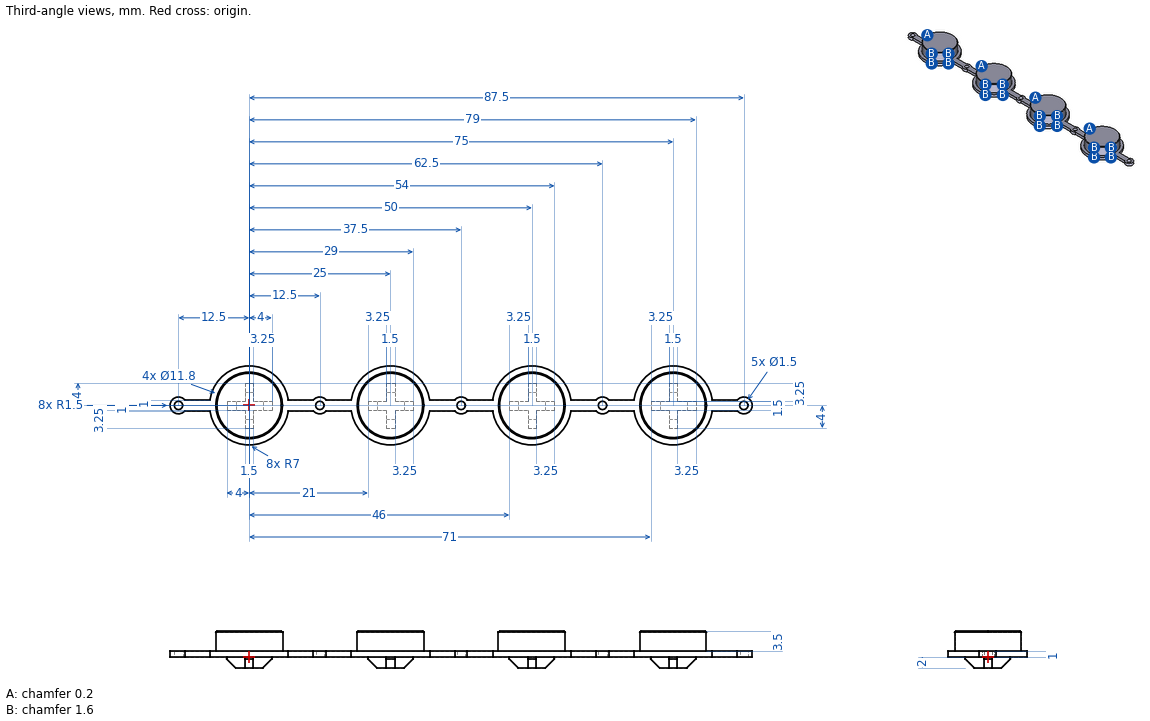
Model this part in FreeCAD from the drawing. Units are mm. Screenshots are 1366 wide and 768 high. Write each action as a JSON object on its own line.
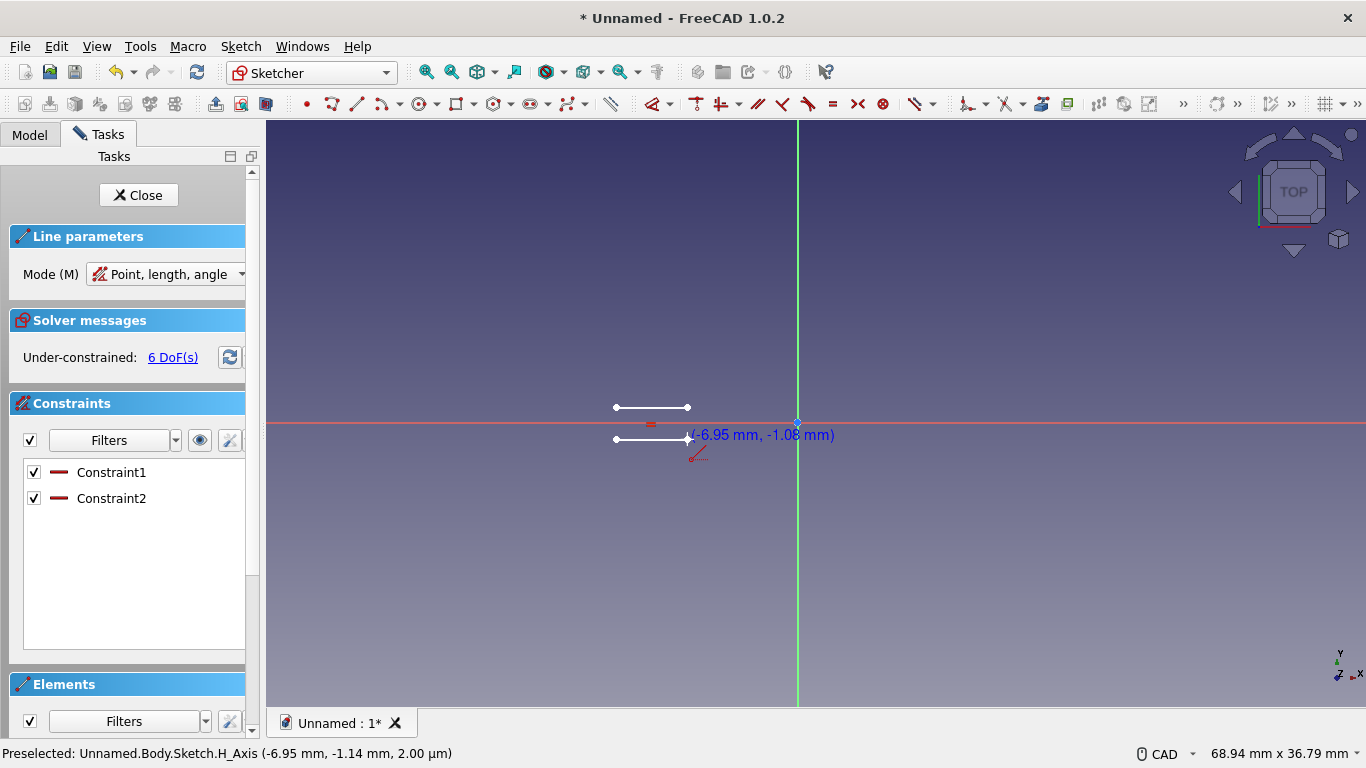
{"action": "left_click", "coordinate": [908, 439]}
{"action": "left_click", "coordinate": [980, 439]}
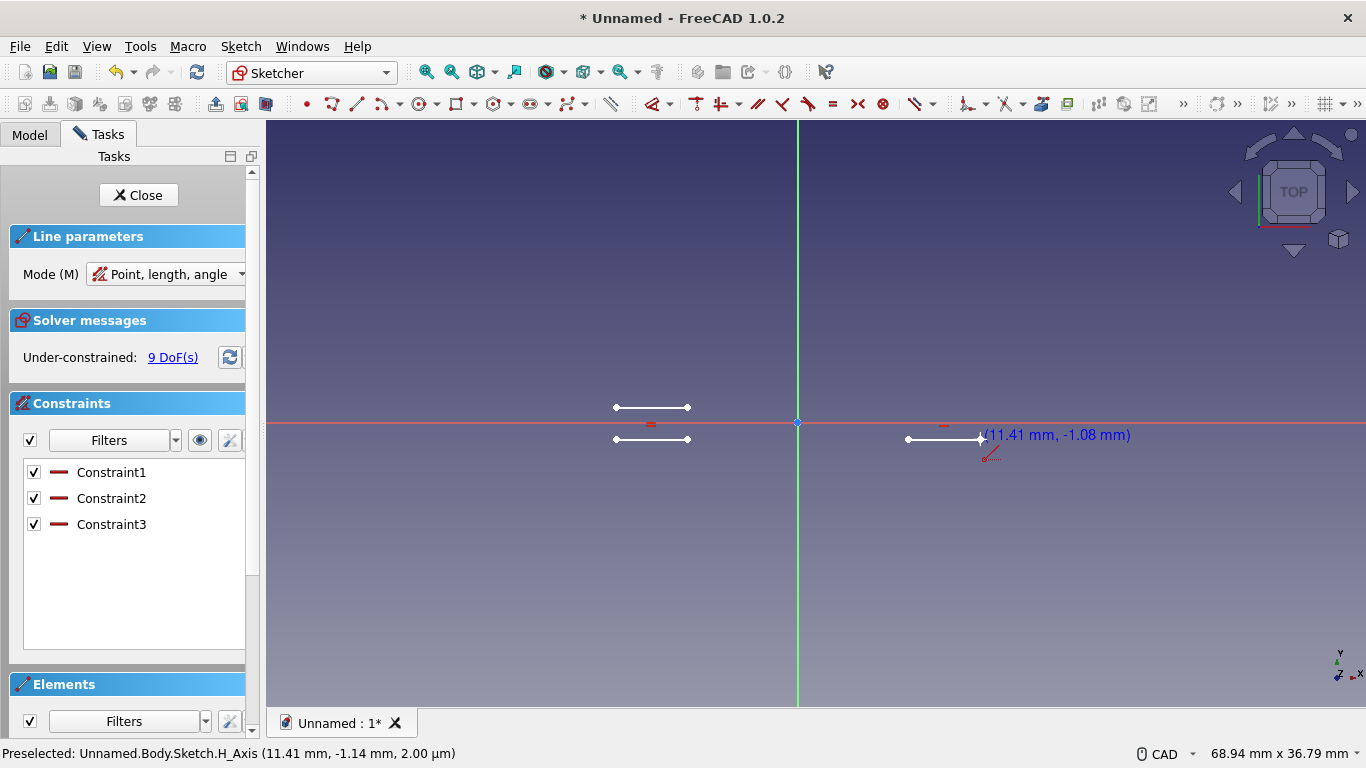
{"action": "left_click", "coordinate": [1015, 439]}
{"action": "left_click", "coordinate": [1086, 439]}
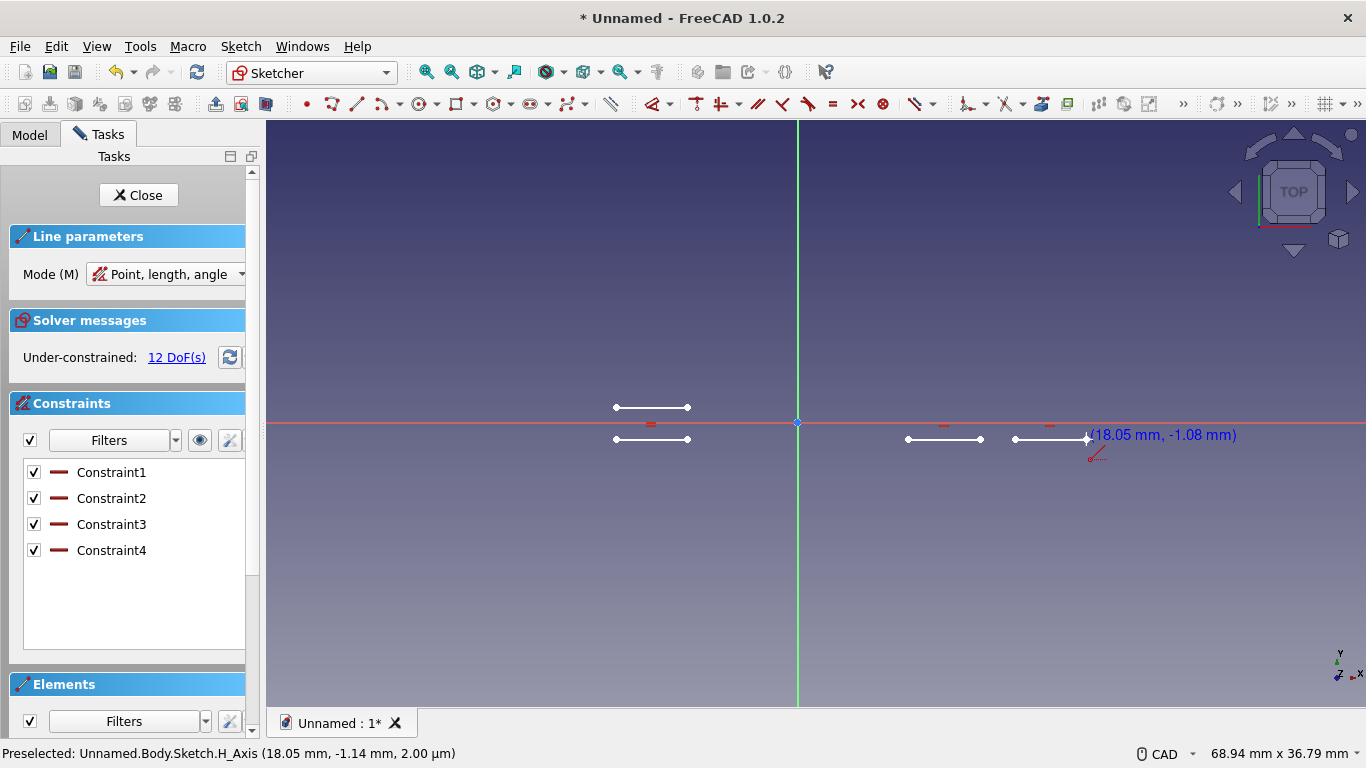
{"action": "scroll", "coordinate": [370, 408], "scroll_direction": "down", "scroll_amount": 5}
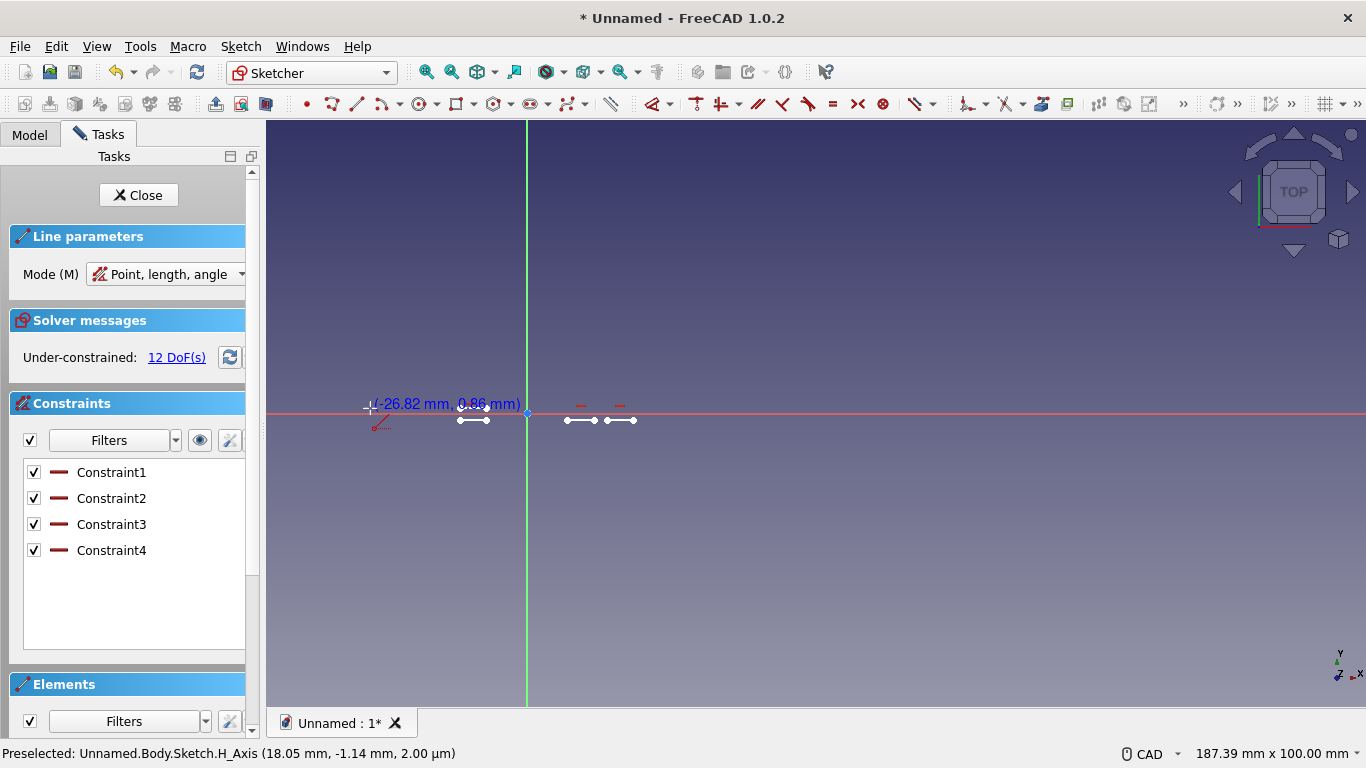
{"action": "scroll", "coordinate": [715, 420], "scroll_direction": "up", "scroll_amount": 5}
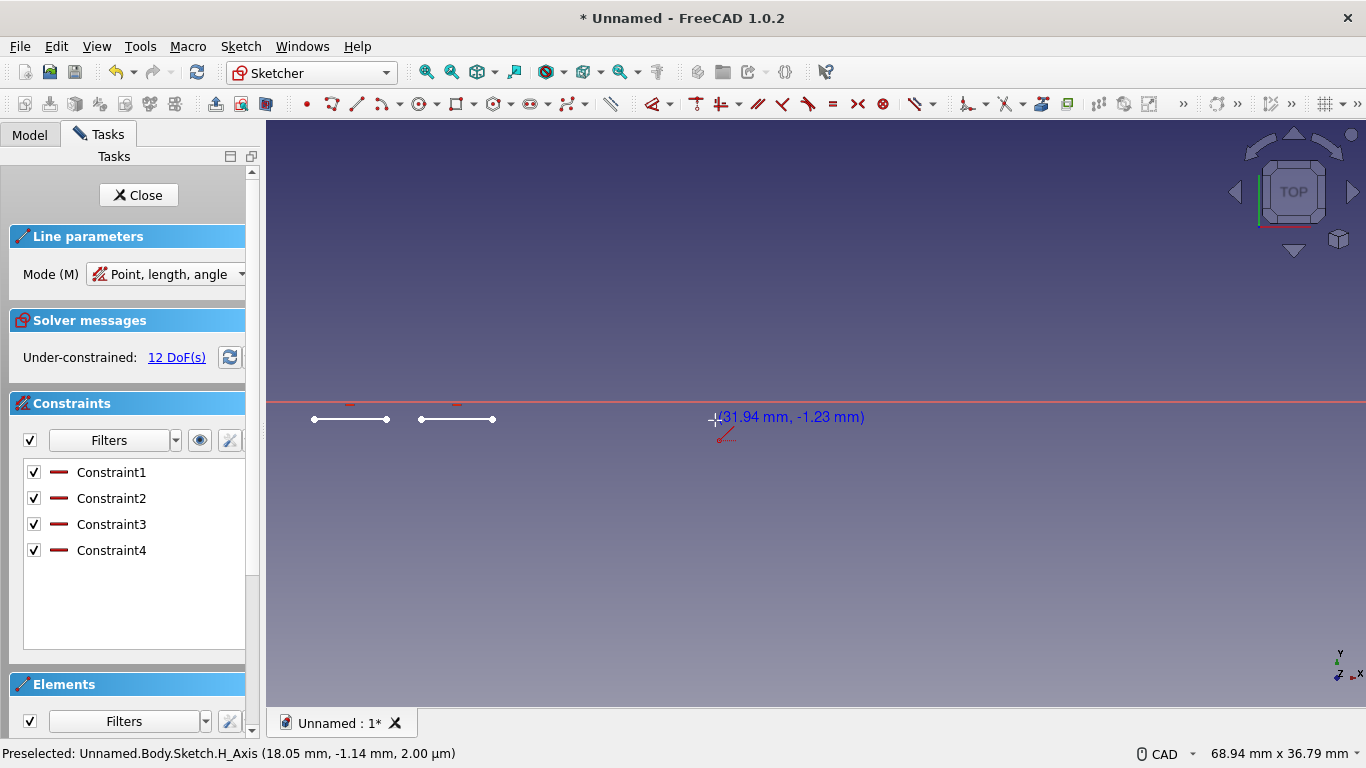
{"action": "left_click", "coordinate": [714, 418]}
{"action": "left_click", "coordinate": [785, 418]}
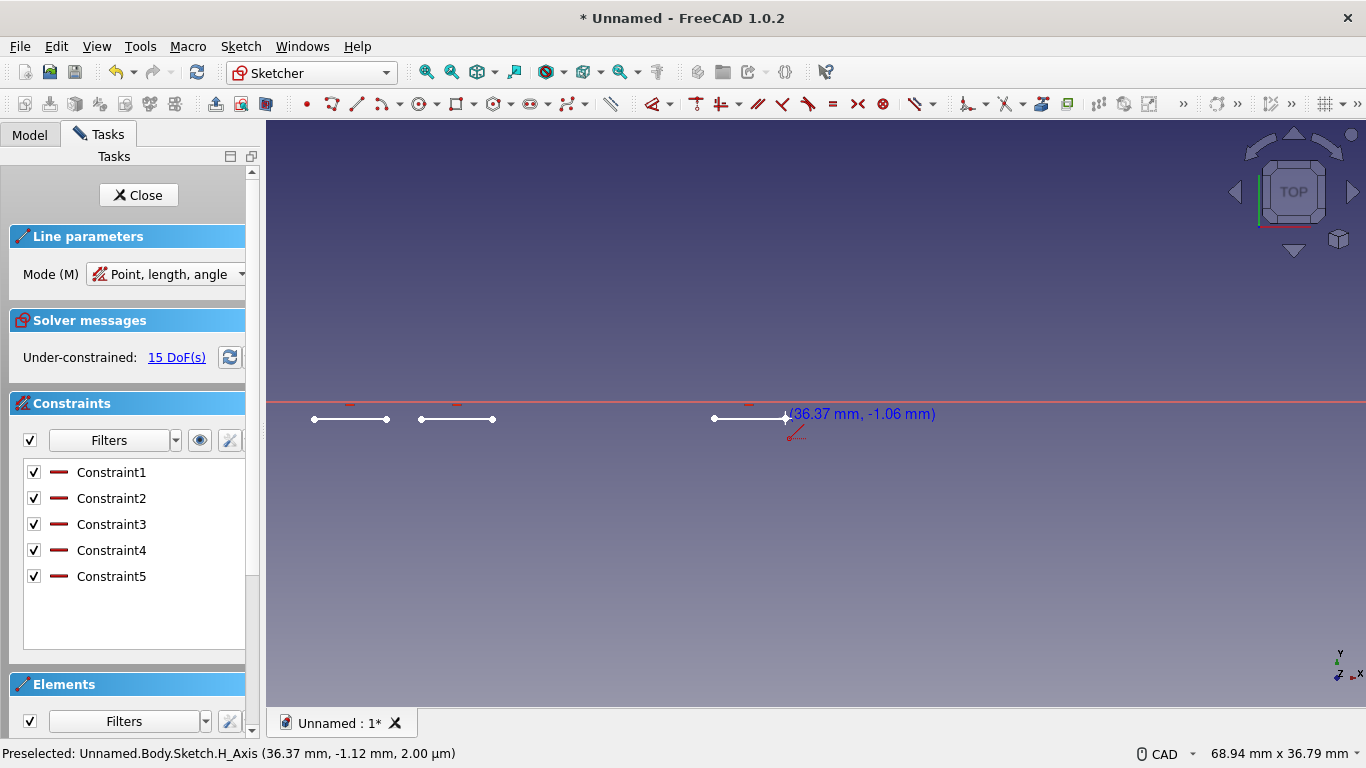
{"action": "left_click", "coordinate": [821, 418]}
{"action": "left_click", "coordinate": [892, 418]}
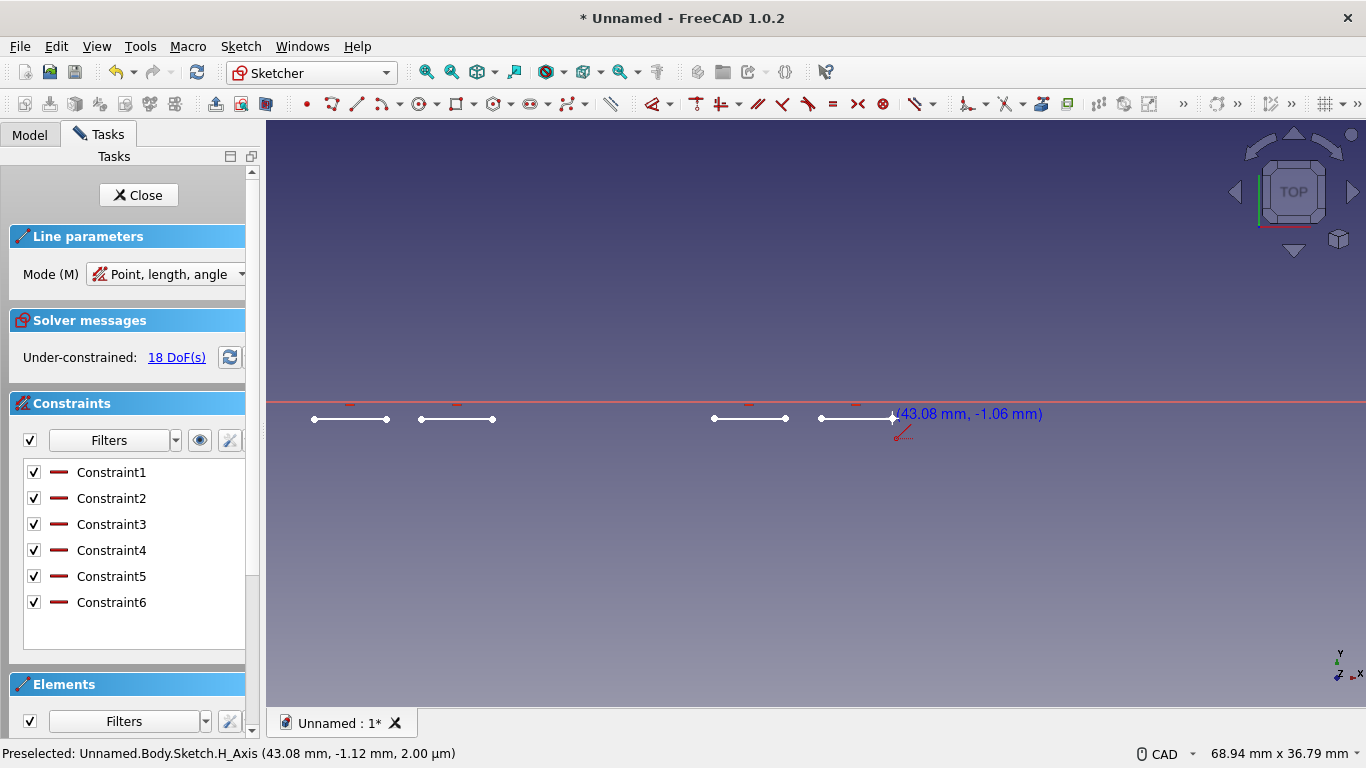
{"action": "left_click", "coordinate": [1113, 418]}
{"action": "left_click", "coordinate": [1184, 418]}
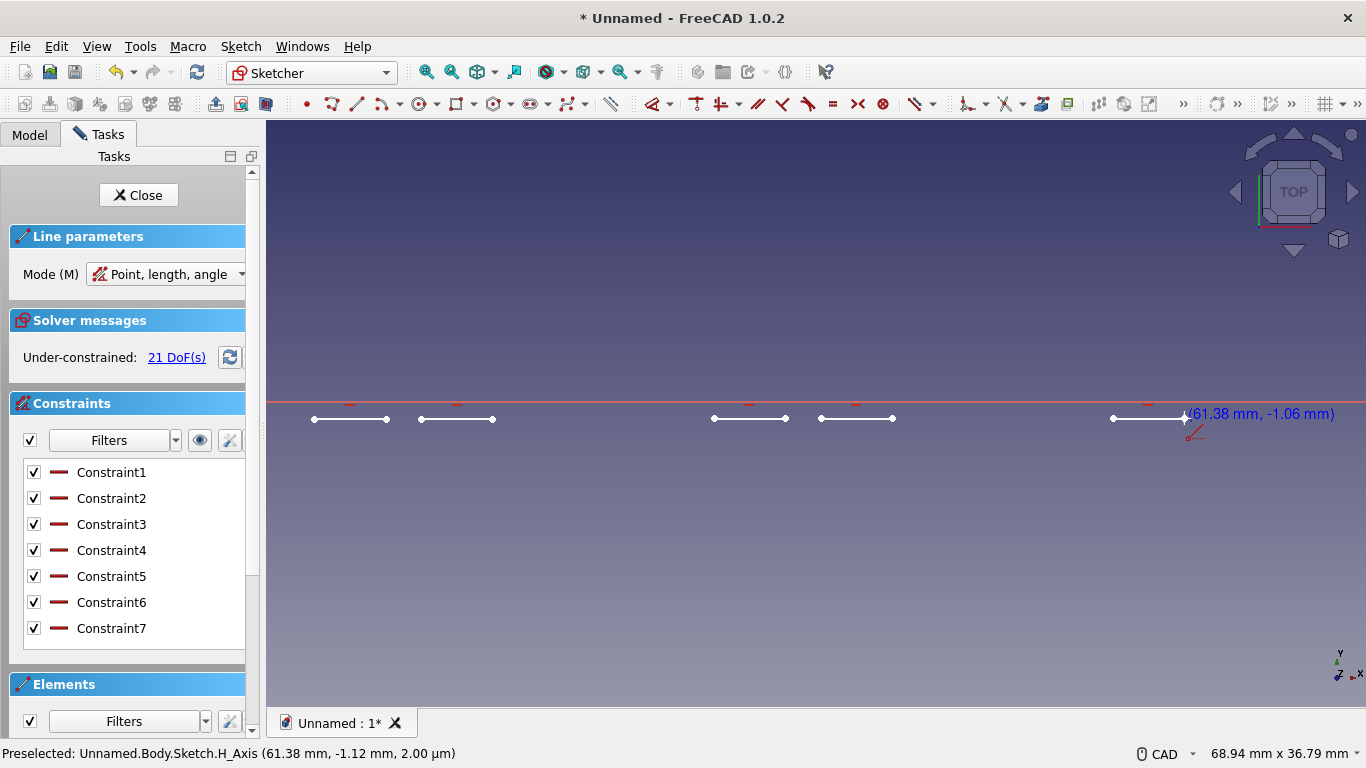
{"action": "scroll", "coordinate": [715, 420], "scroll_direction": "down", "scroll_amount": 5}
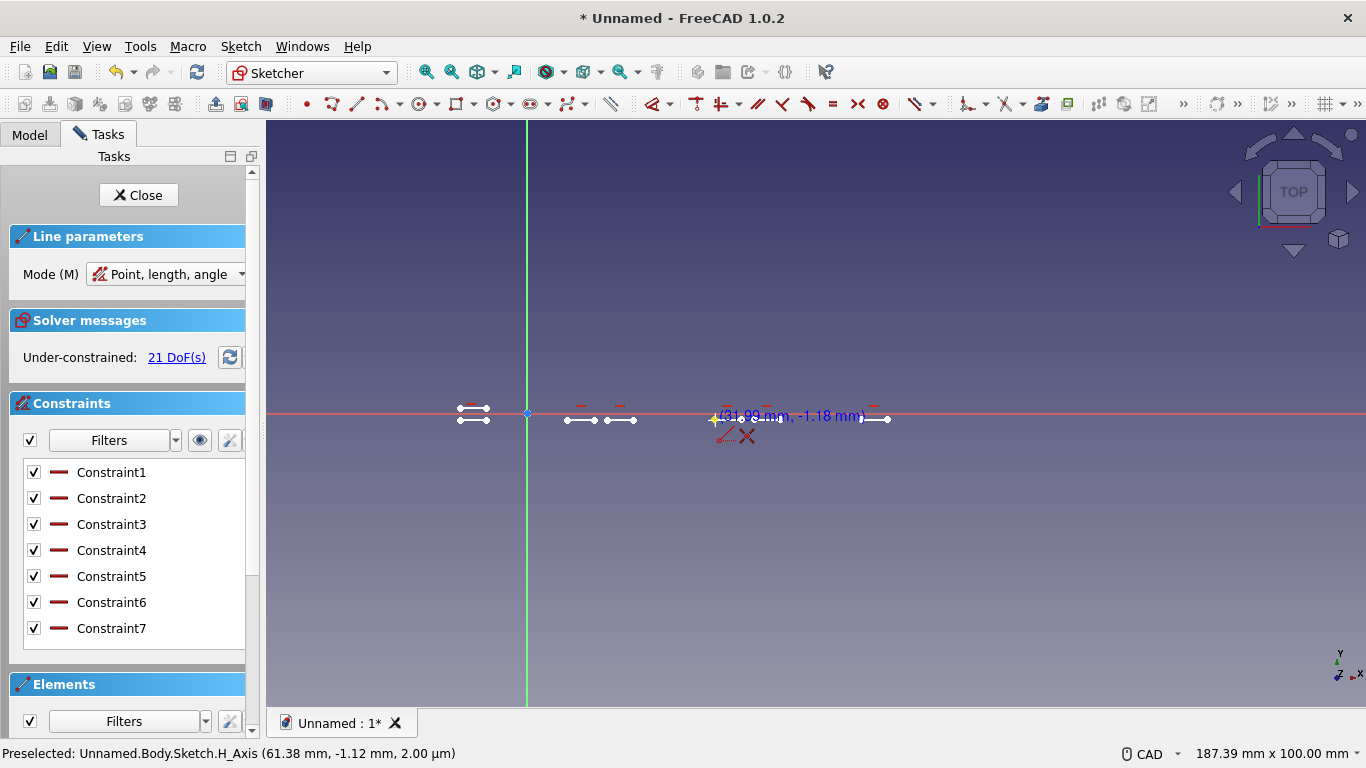
{"action": "scroll", "coordinate": [901, 420], "scroll_direction": "up", "scroll_amount": 5}